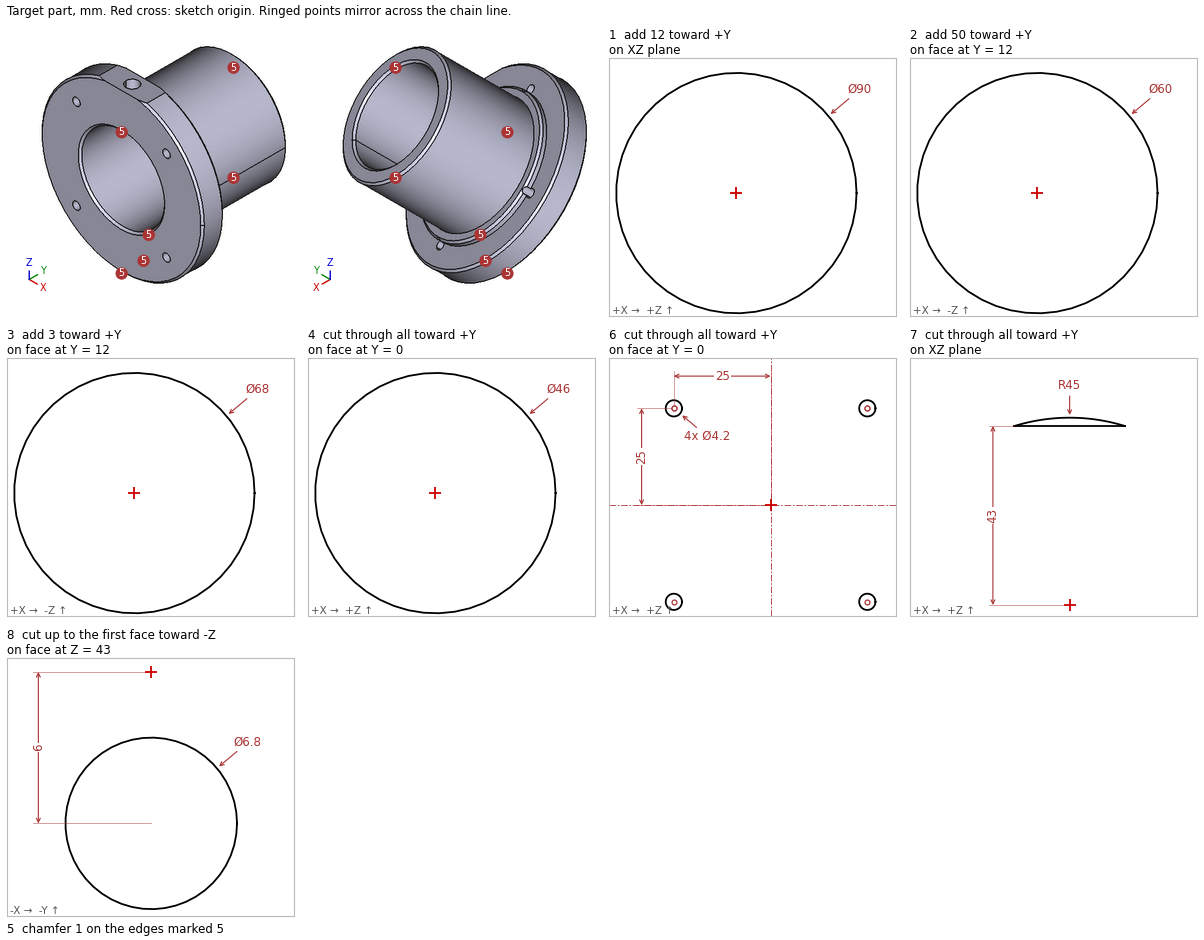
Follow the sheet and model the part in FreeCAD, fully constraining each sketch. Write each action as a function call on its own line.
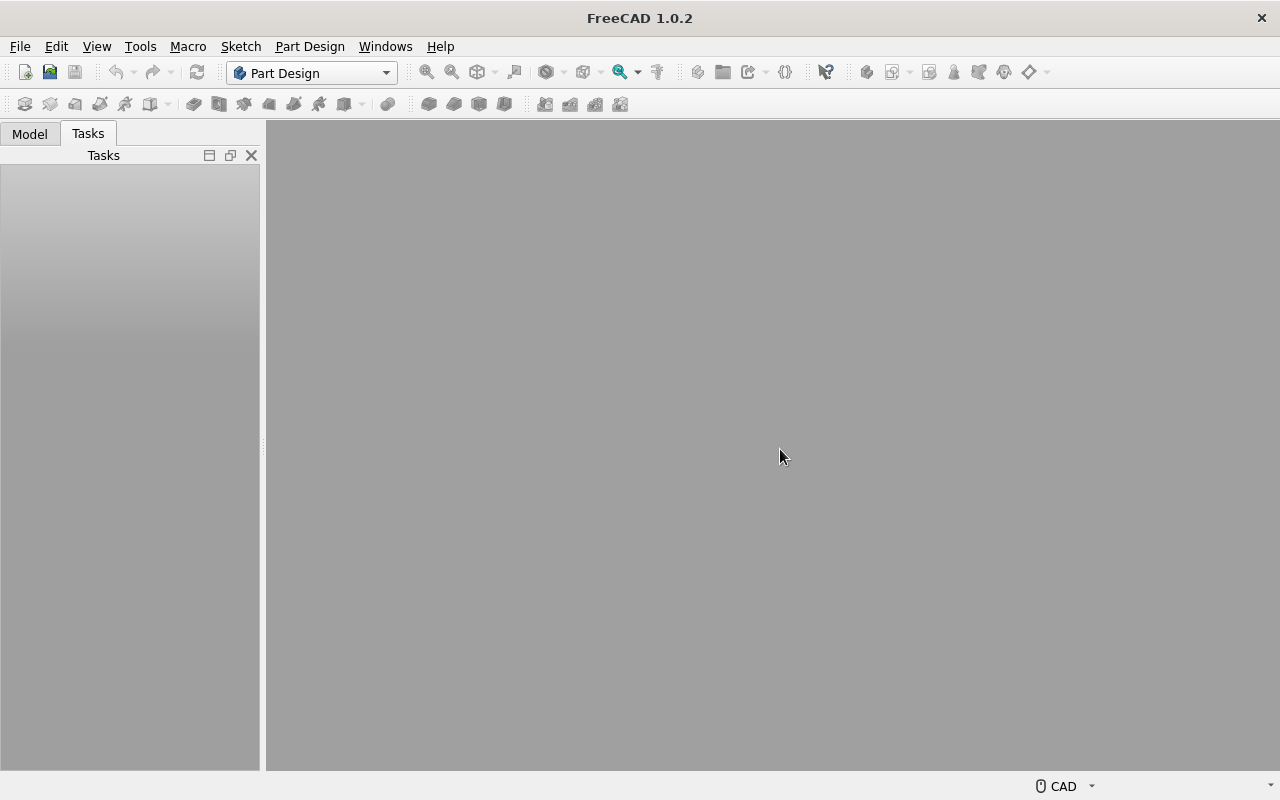
click(25, 72)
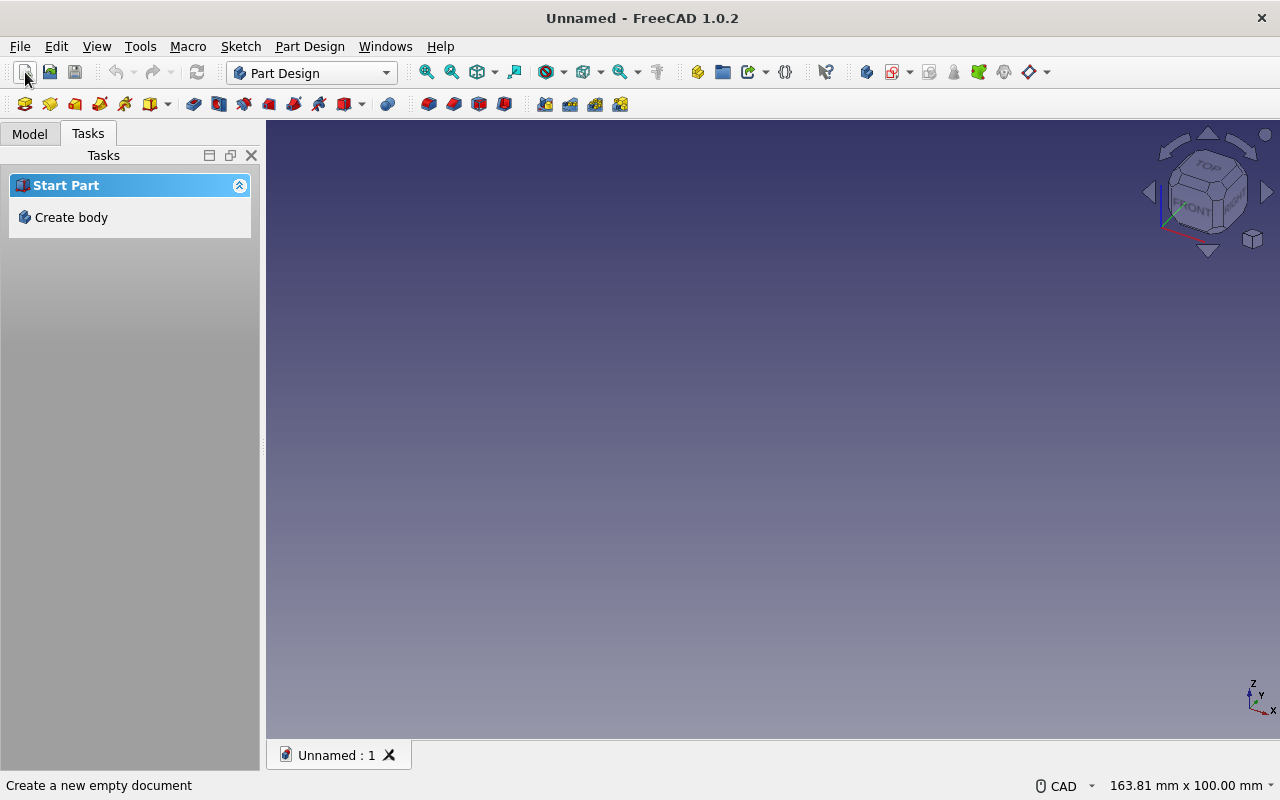
click(892, 72)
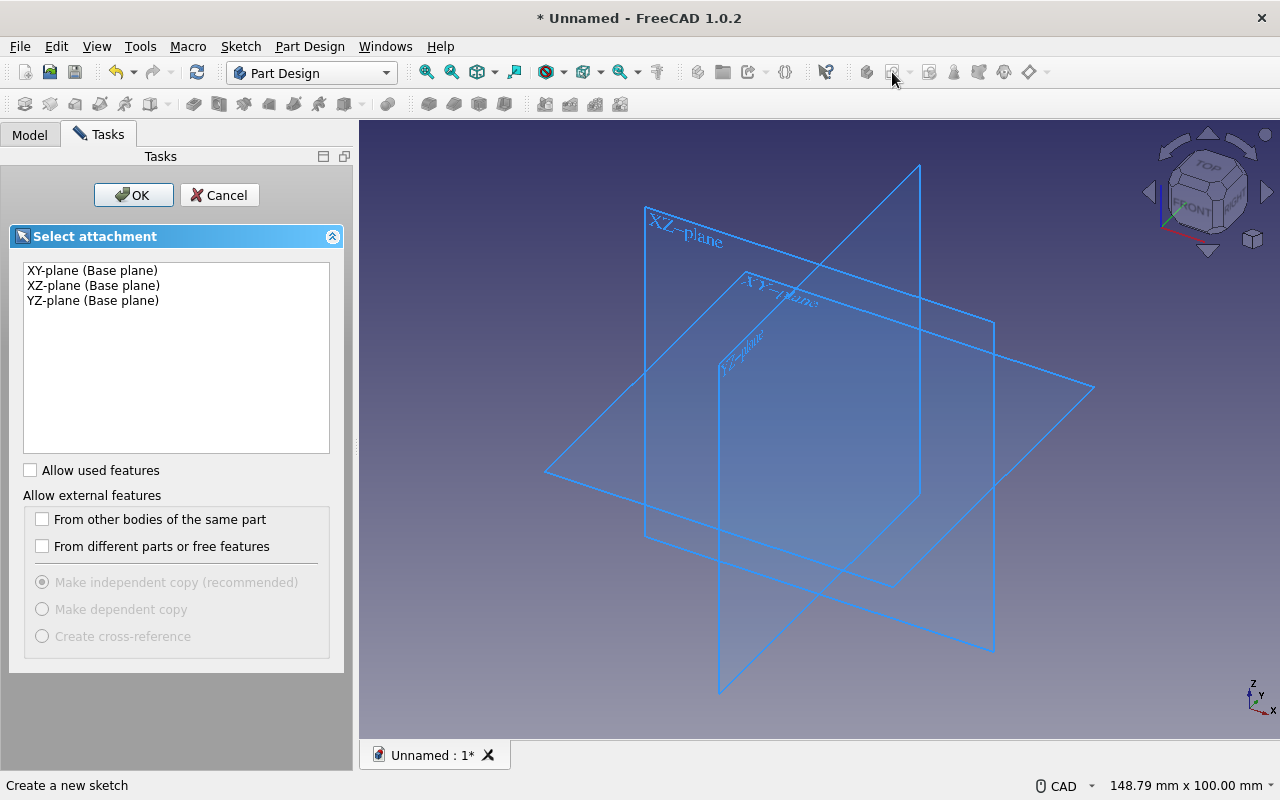
click(84, 286)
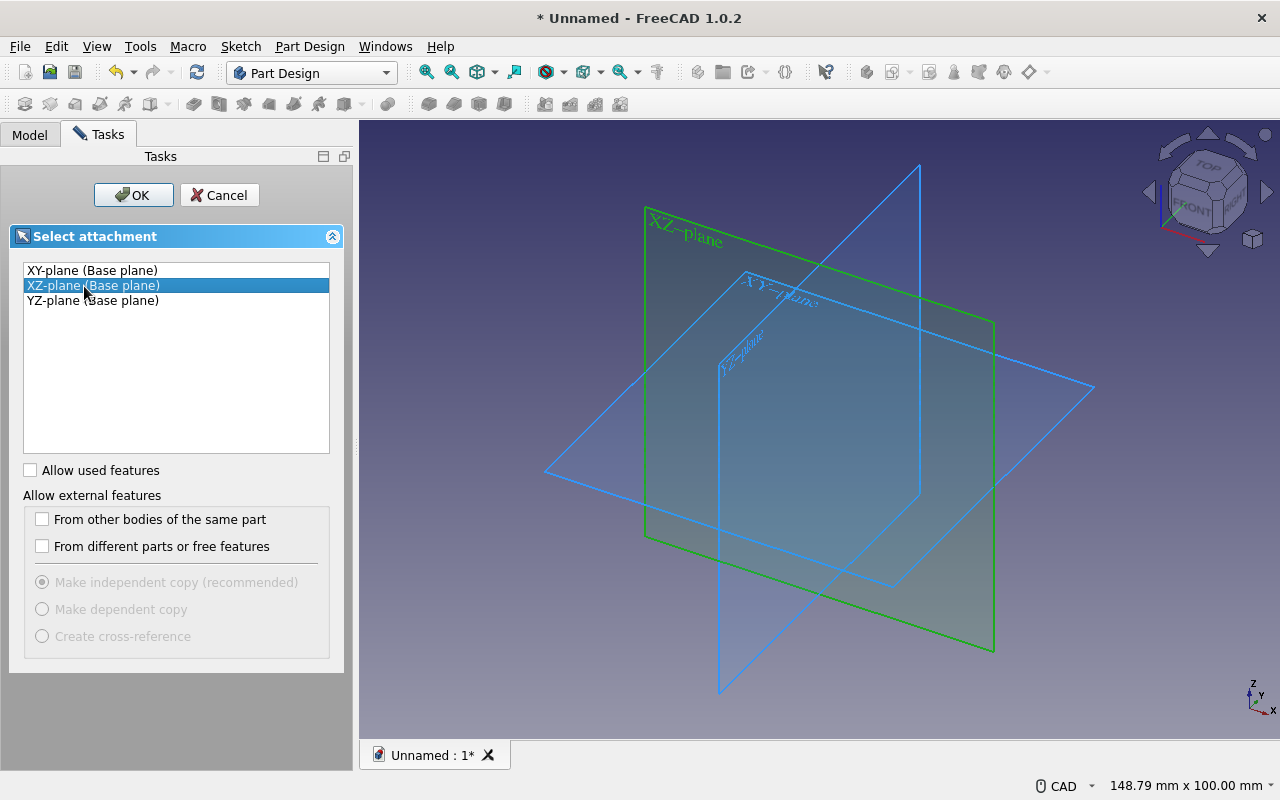
click(134, 195)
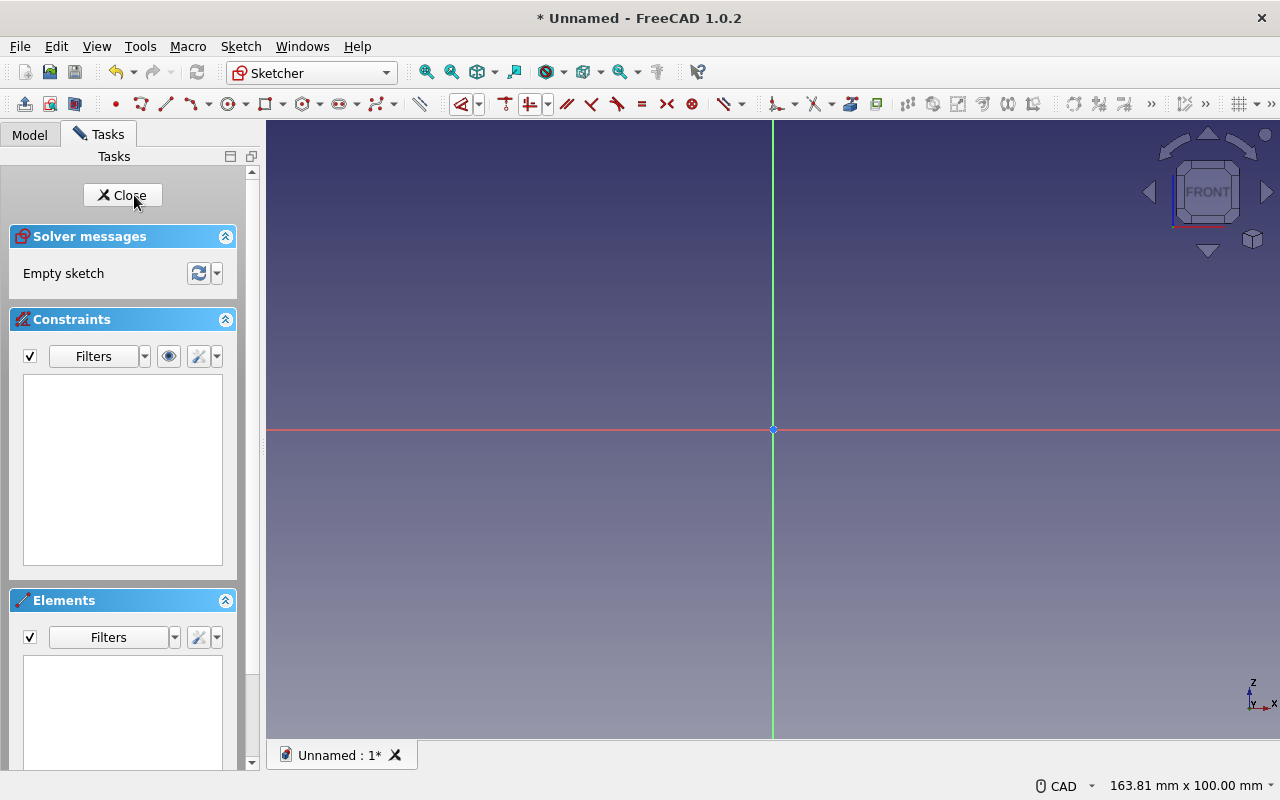
scroll(565, 429, down, 2)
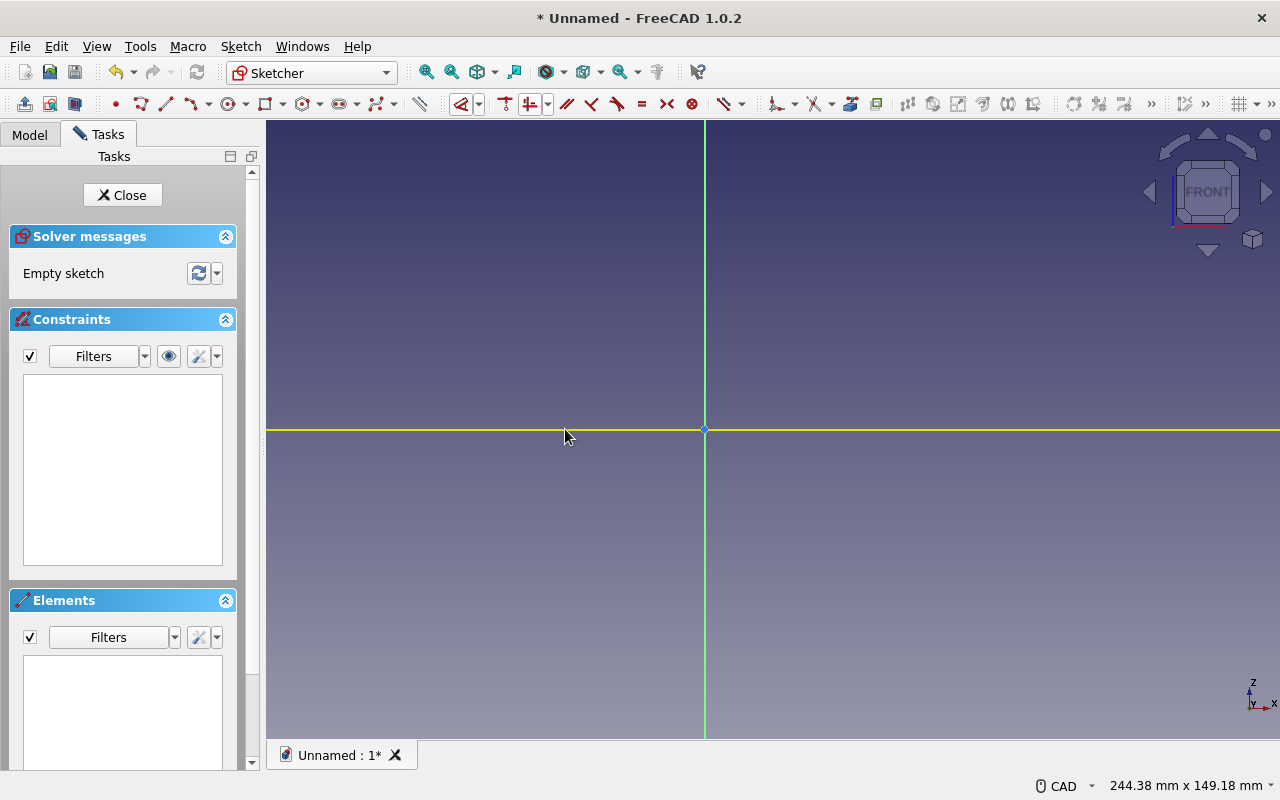
click(228, 104)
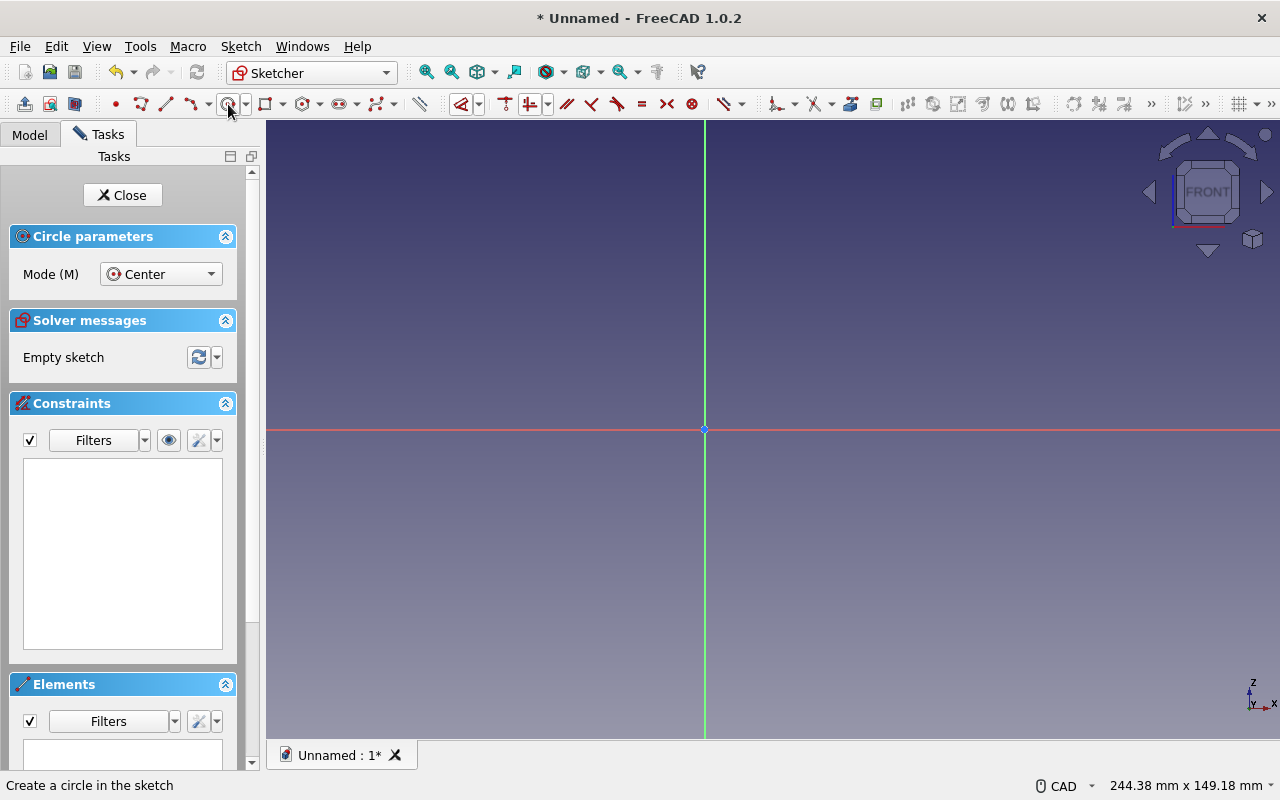
click(705, 430)
move(837, 297)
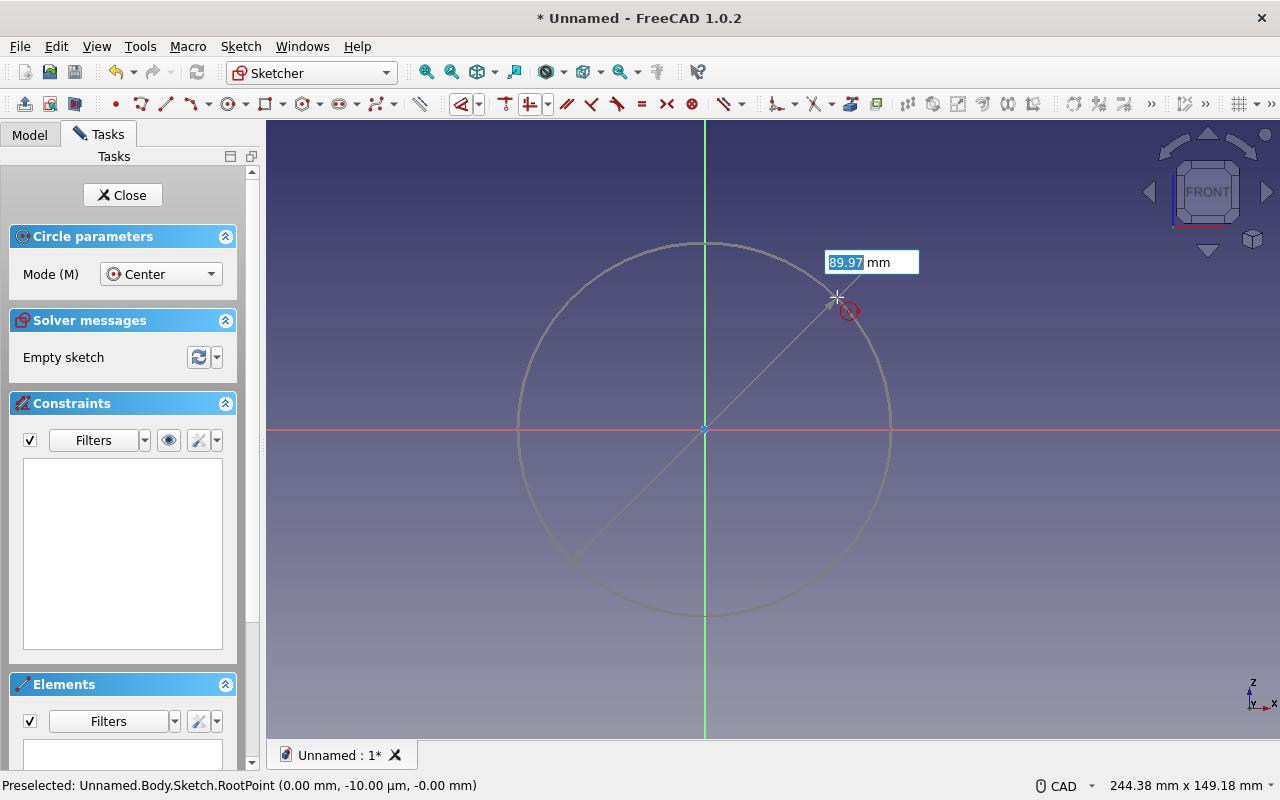
text(90)
key(Return)
key(Escape)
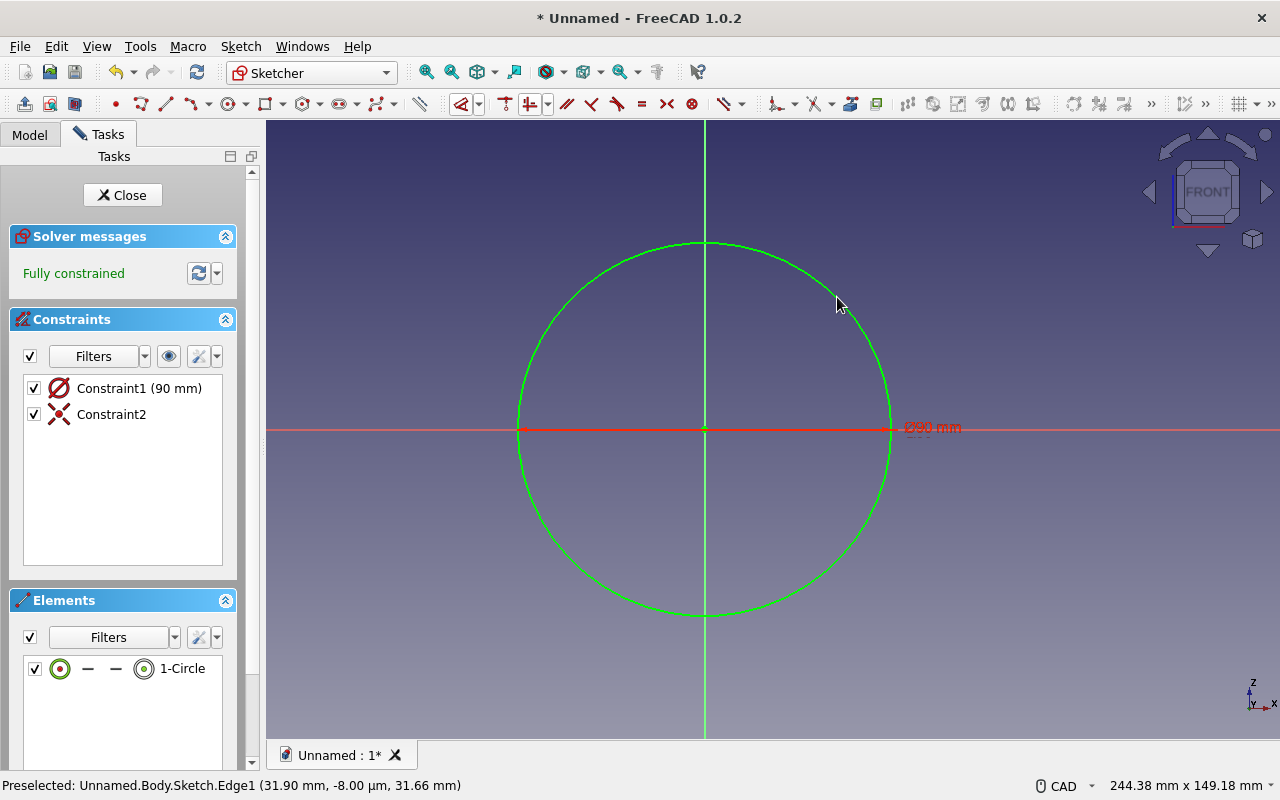
click(123, 195)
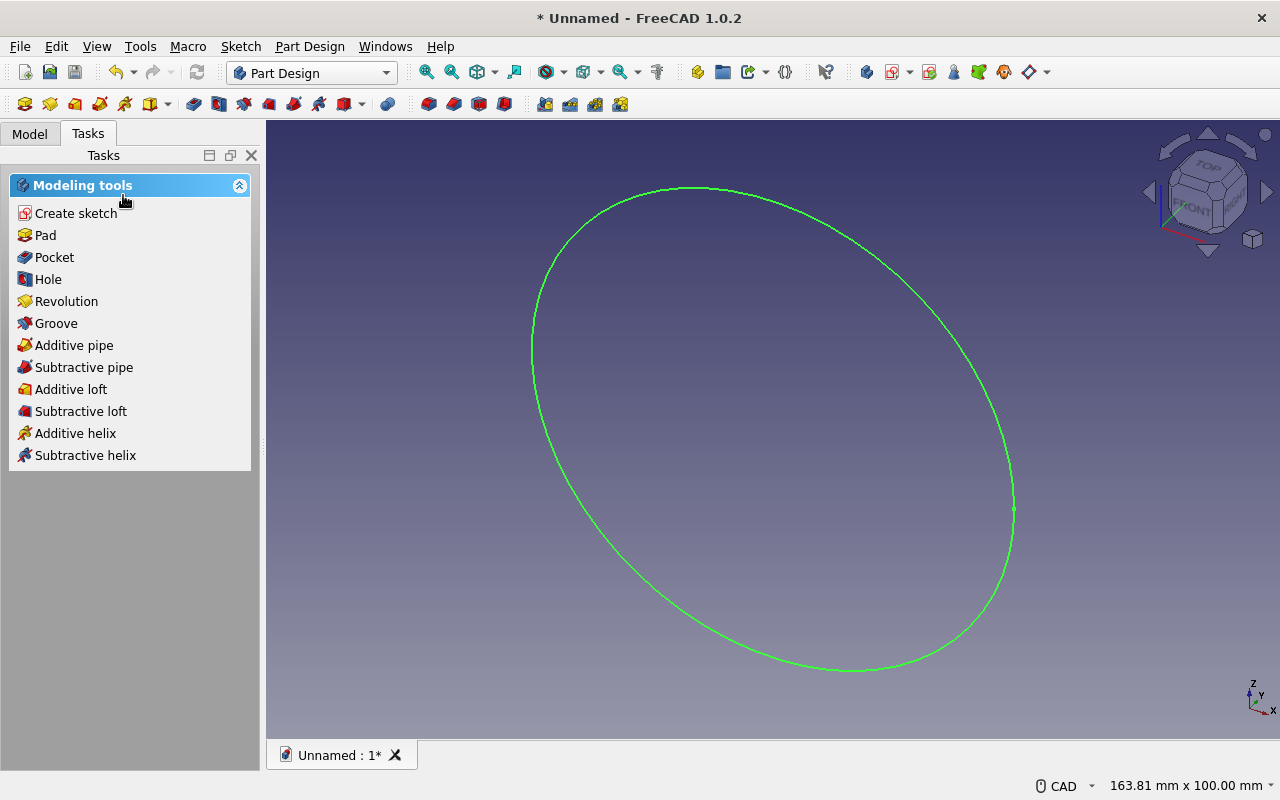
click(25, 104)